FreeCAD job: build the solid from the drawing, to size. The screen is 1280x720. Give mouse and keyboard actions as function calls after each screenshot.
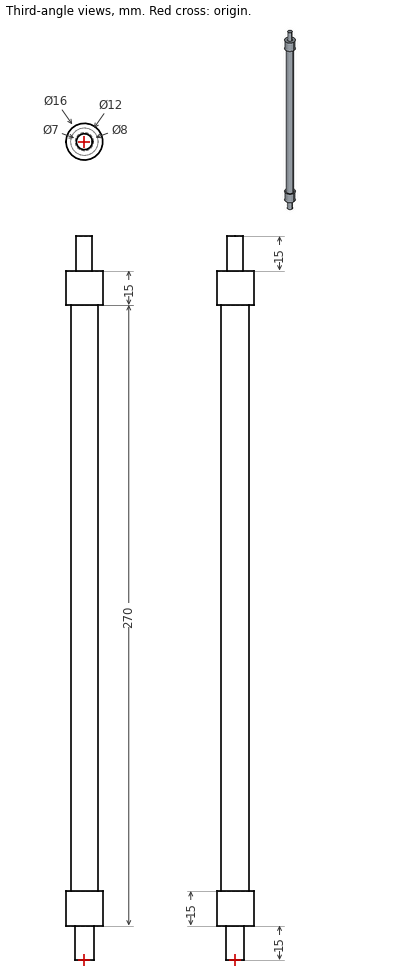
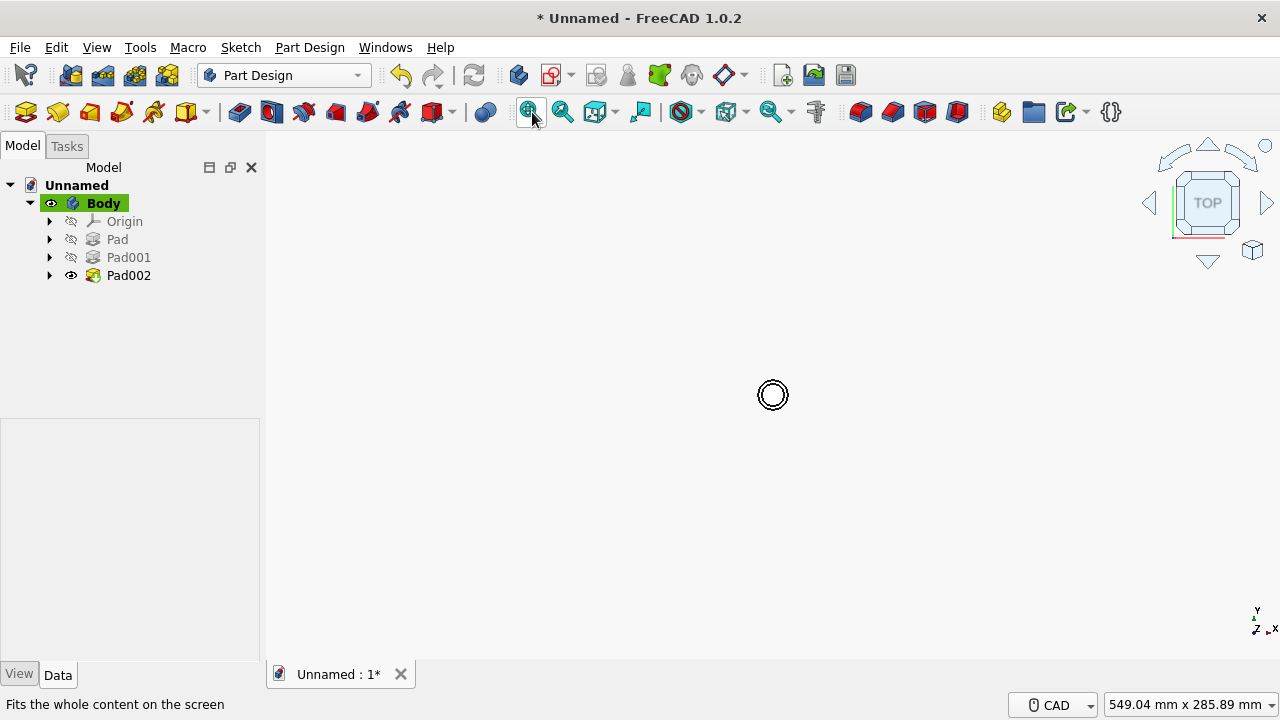
click(532, 112)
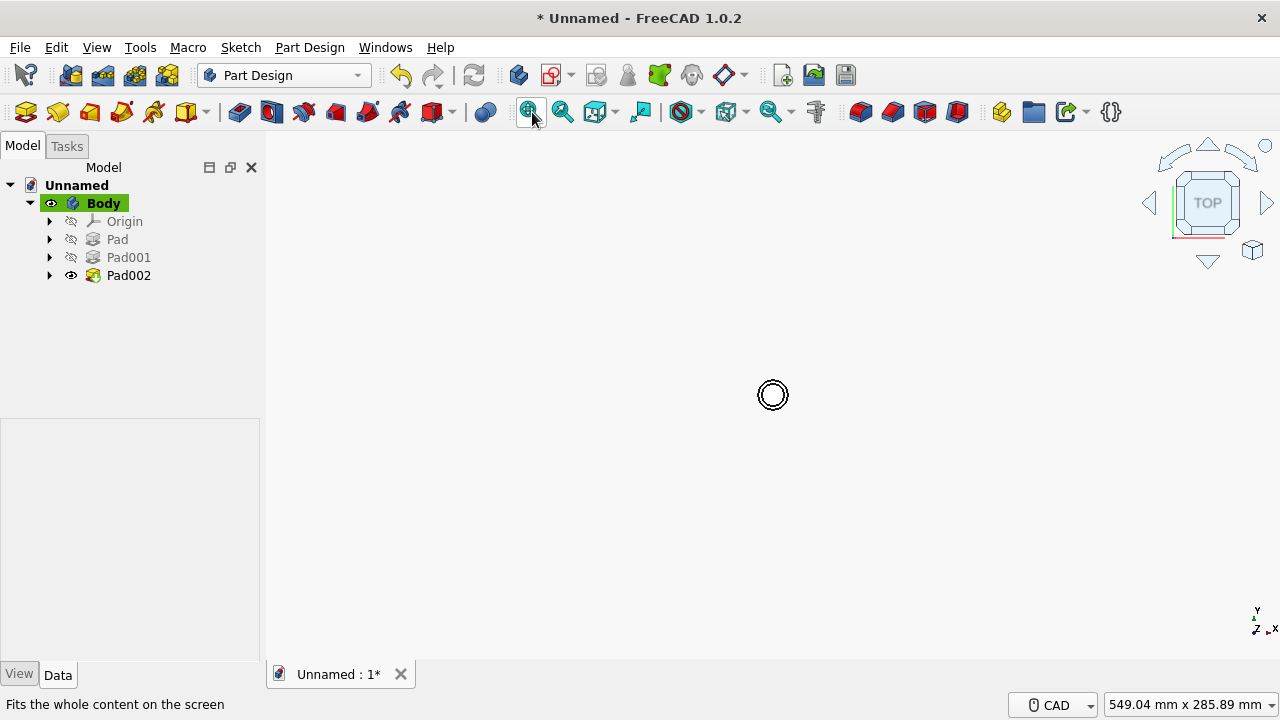
click(773, 394)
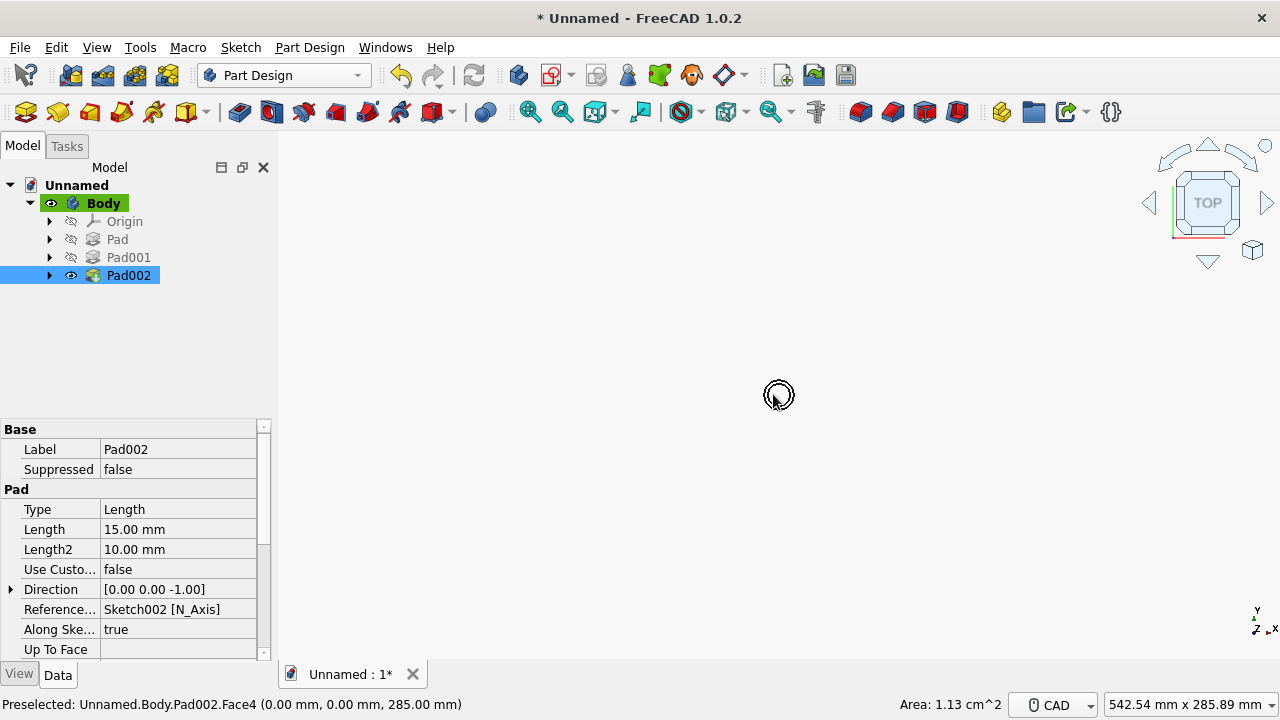
click(552, 76)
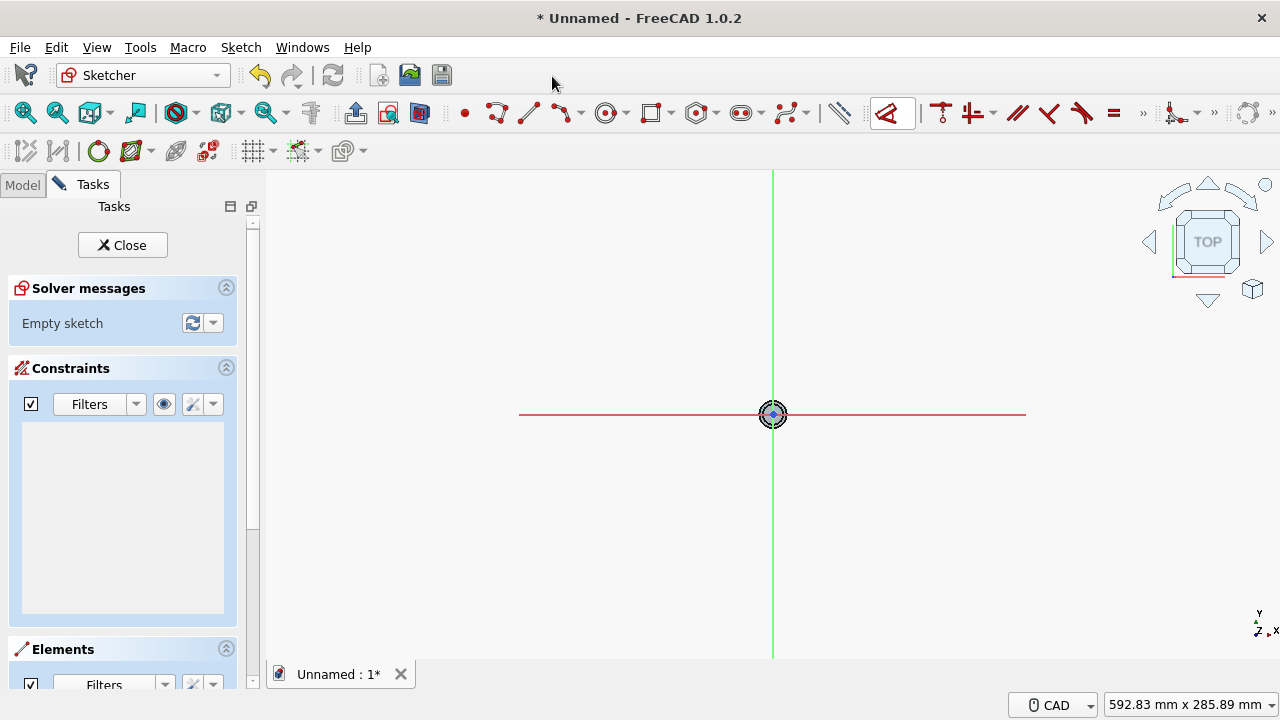
scroll(780, 414, up, 12)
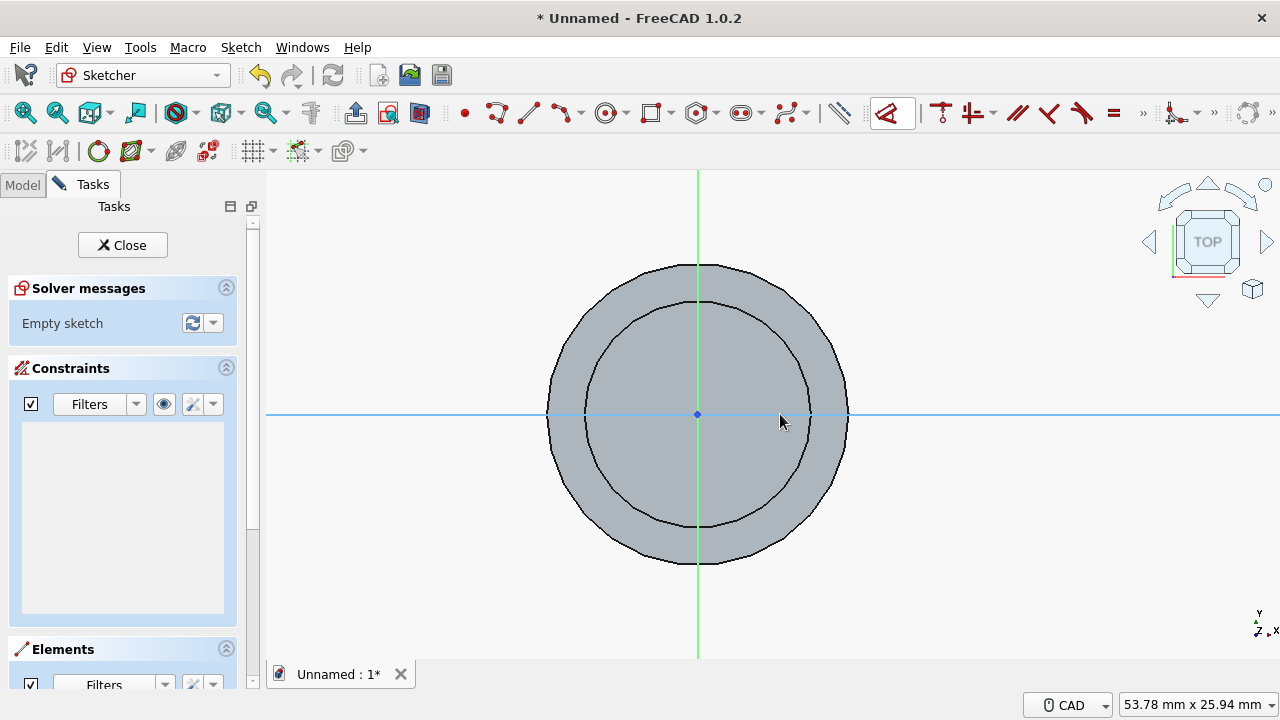
click(606, 114)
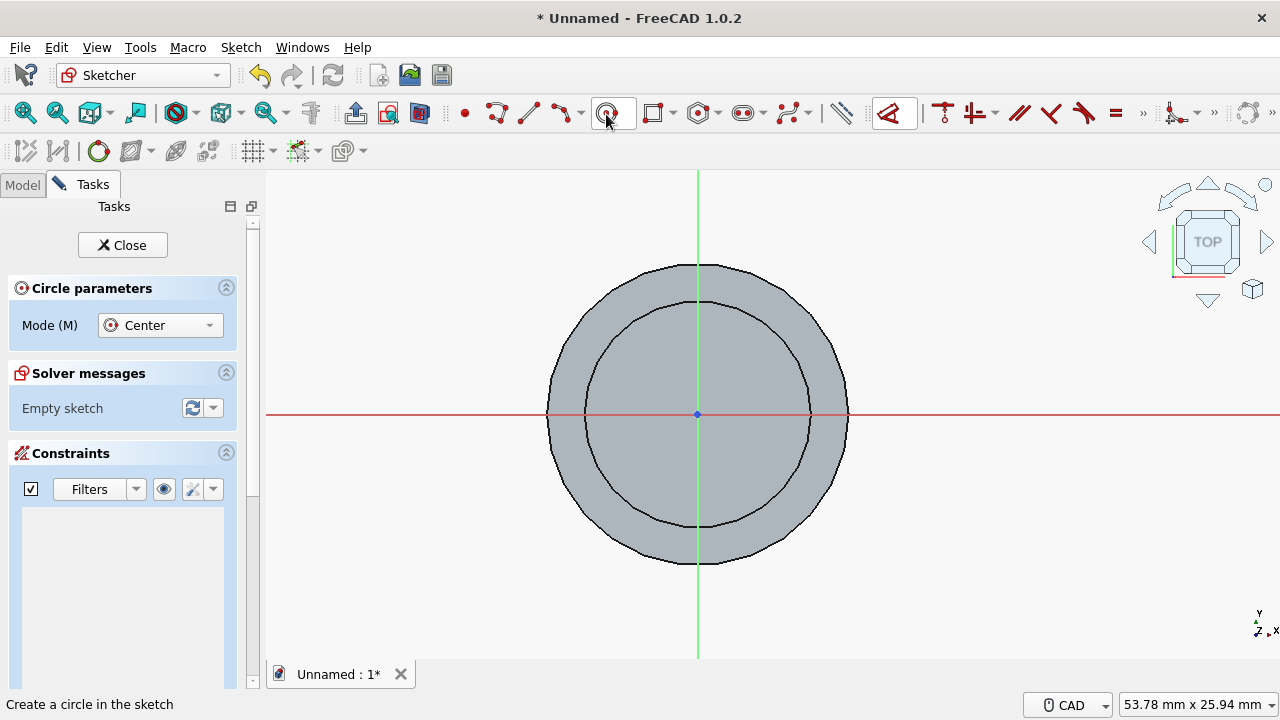
click(698, 414)
click(804, 308)
key(Escape)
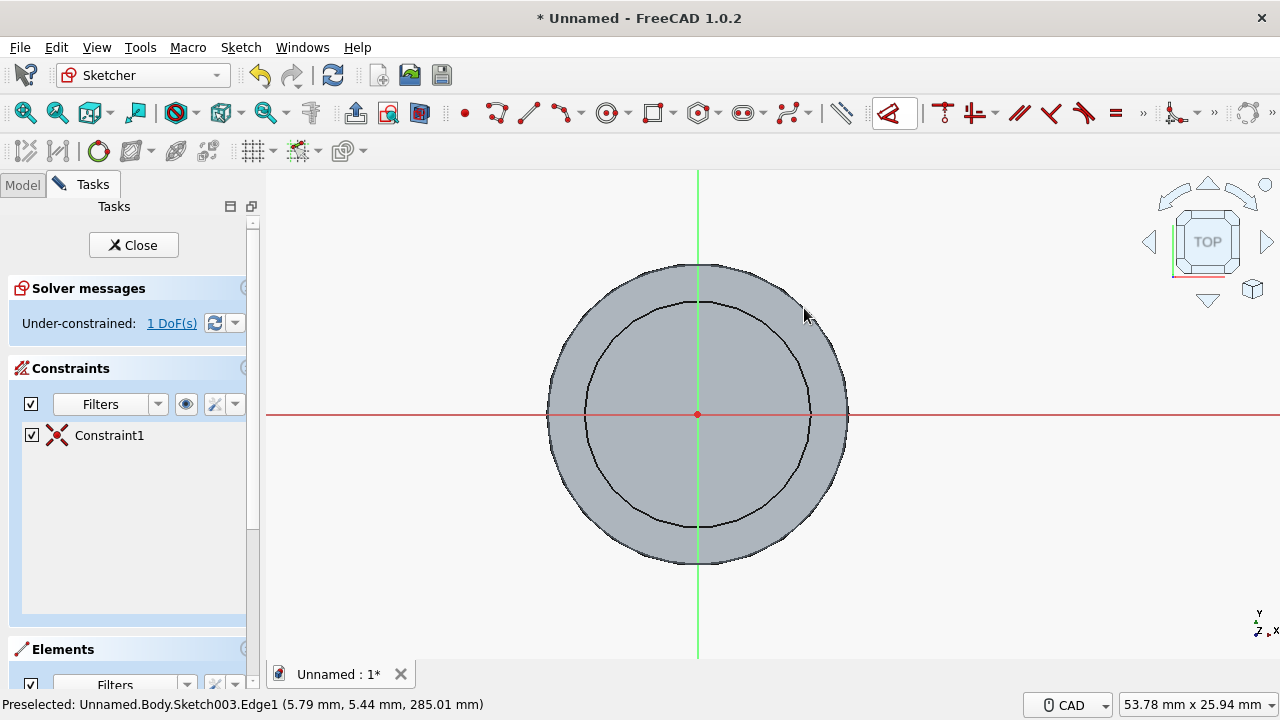
click(803, 308)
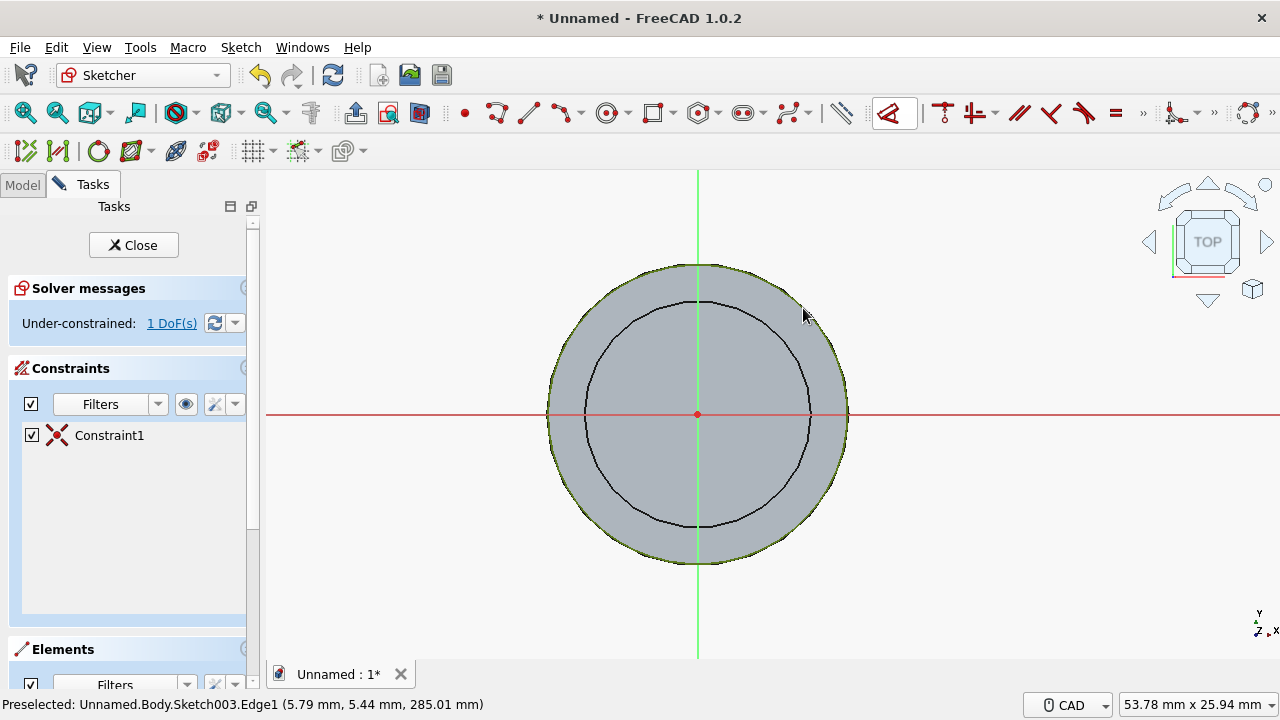
click(912, 114)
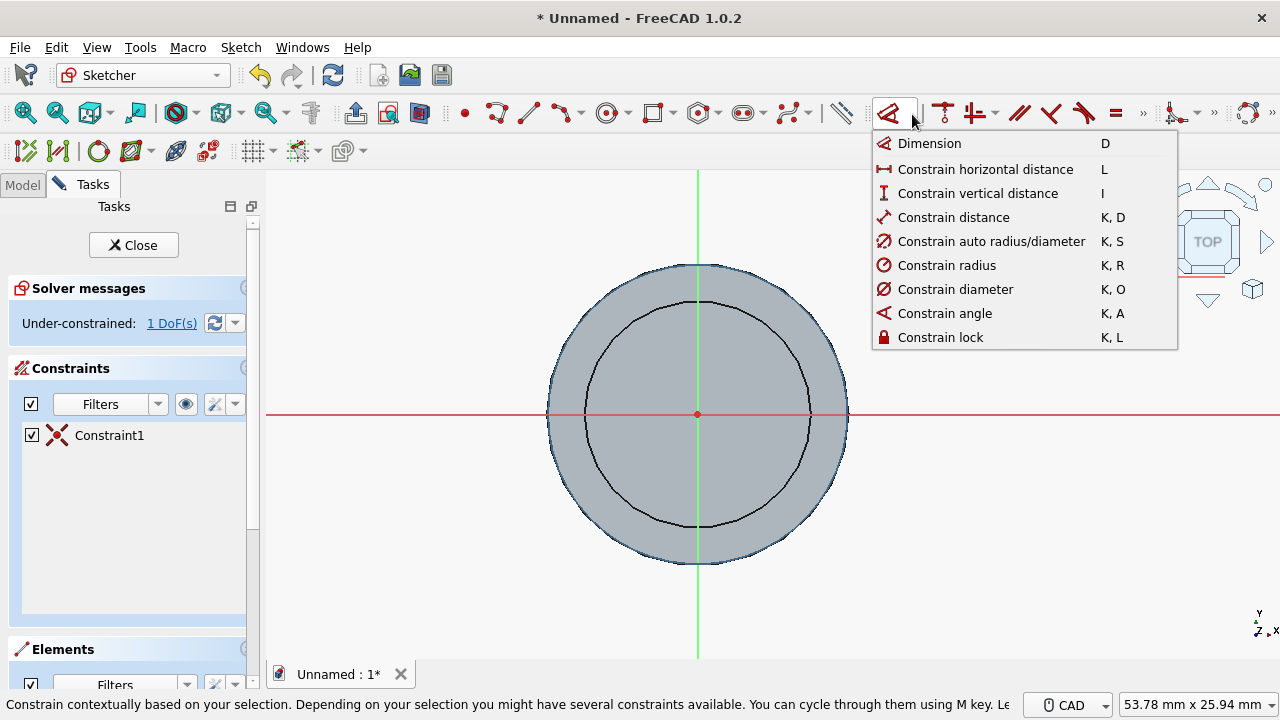
click(1025, 289)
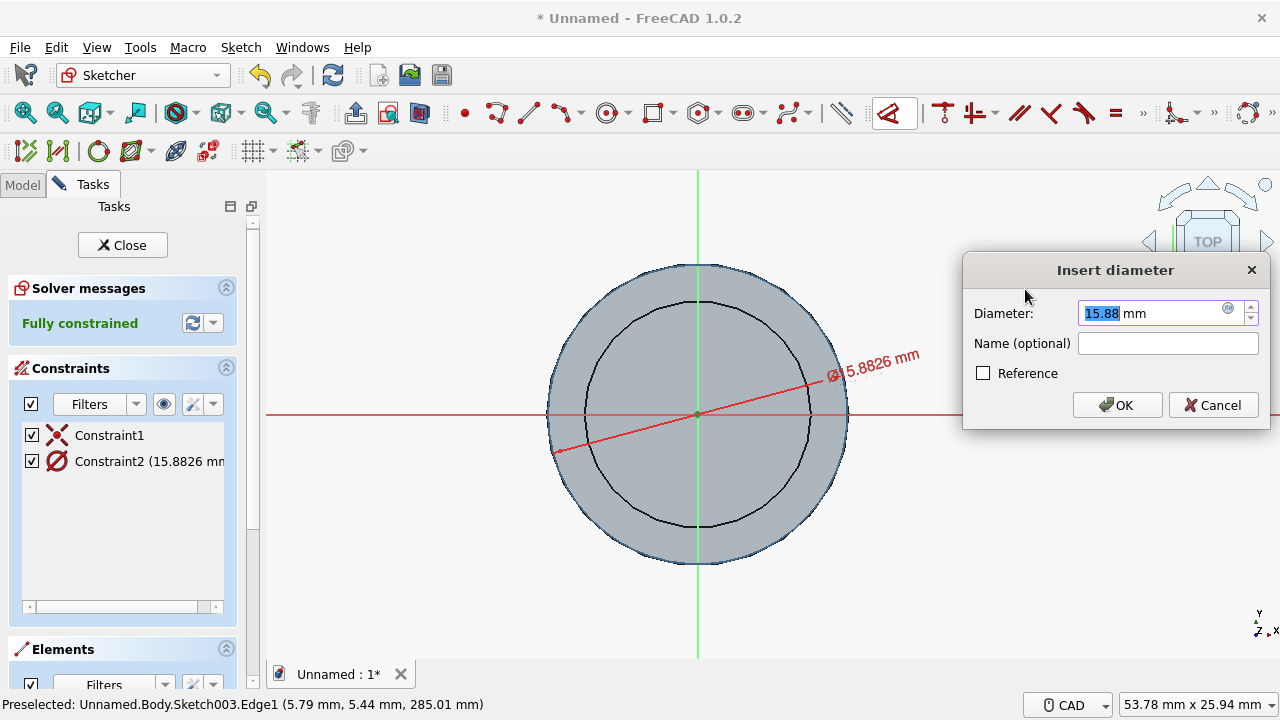
text(16)
key(Return)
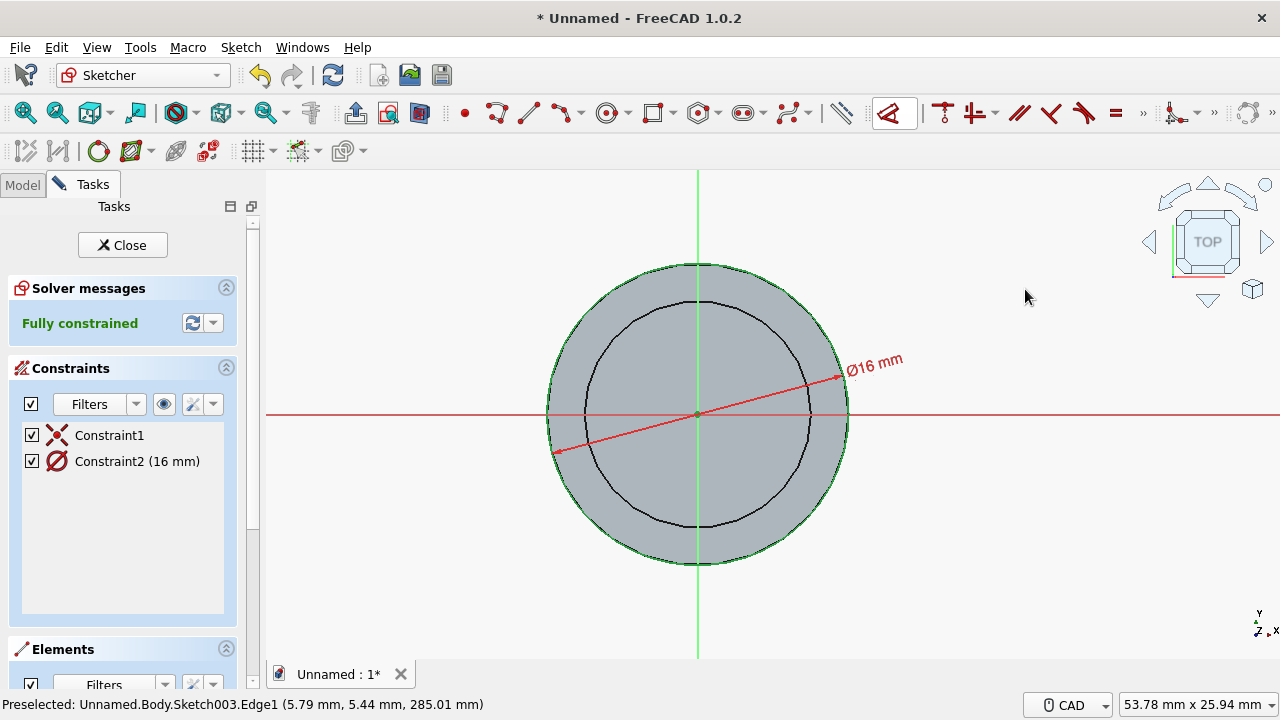
click(123, 245)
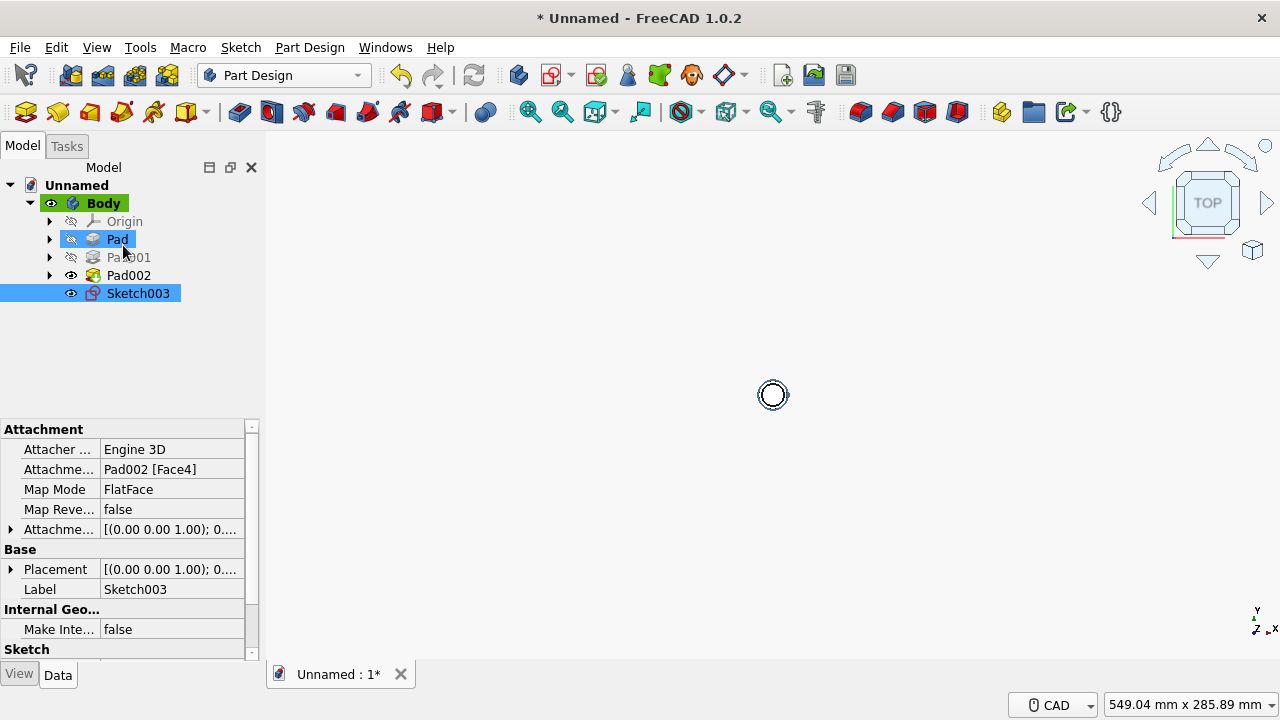
click(26, 112)